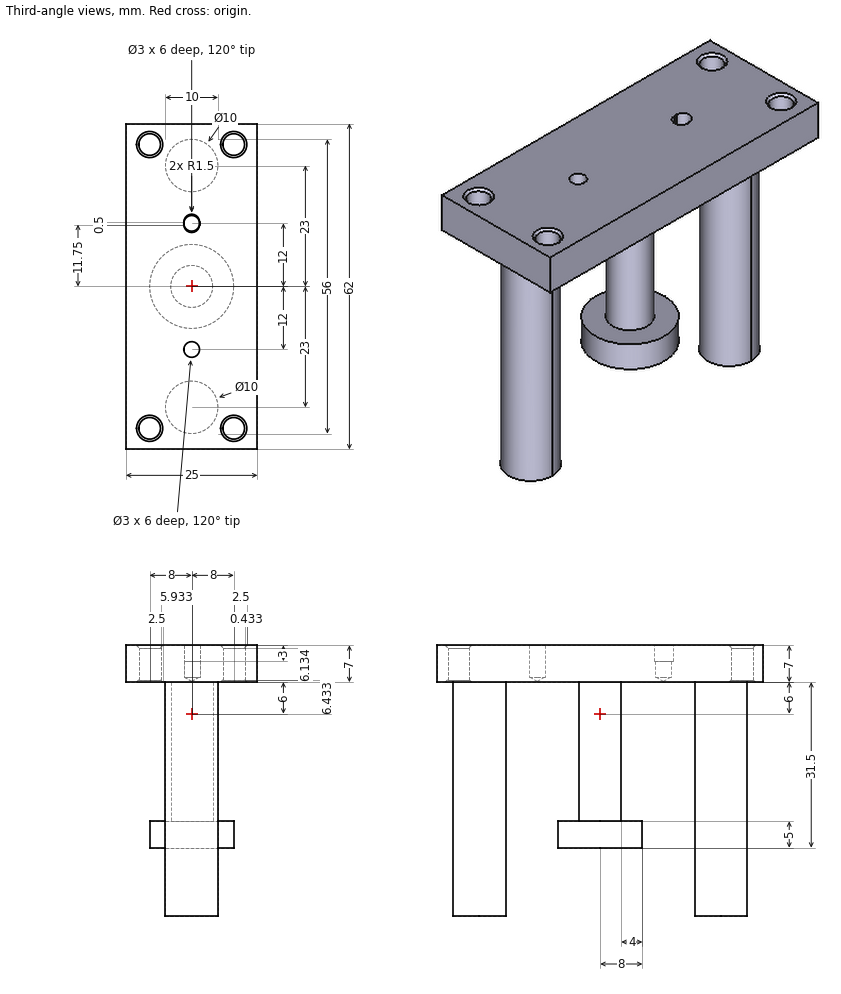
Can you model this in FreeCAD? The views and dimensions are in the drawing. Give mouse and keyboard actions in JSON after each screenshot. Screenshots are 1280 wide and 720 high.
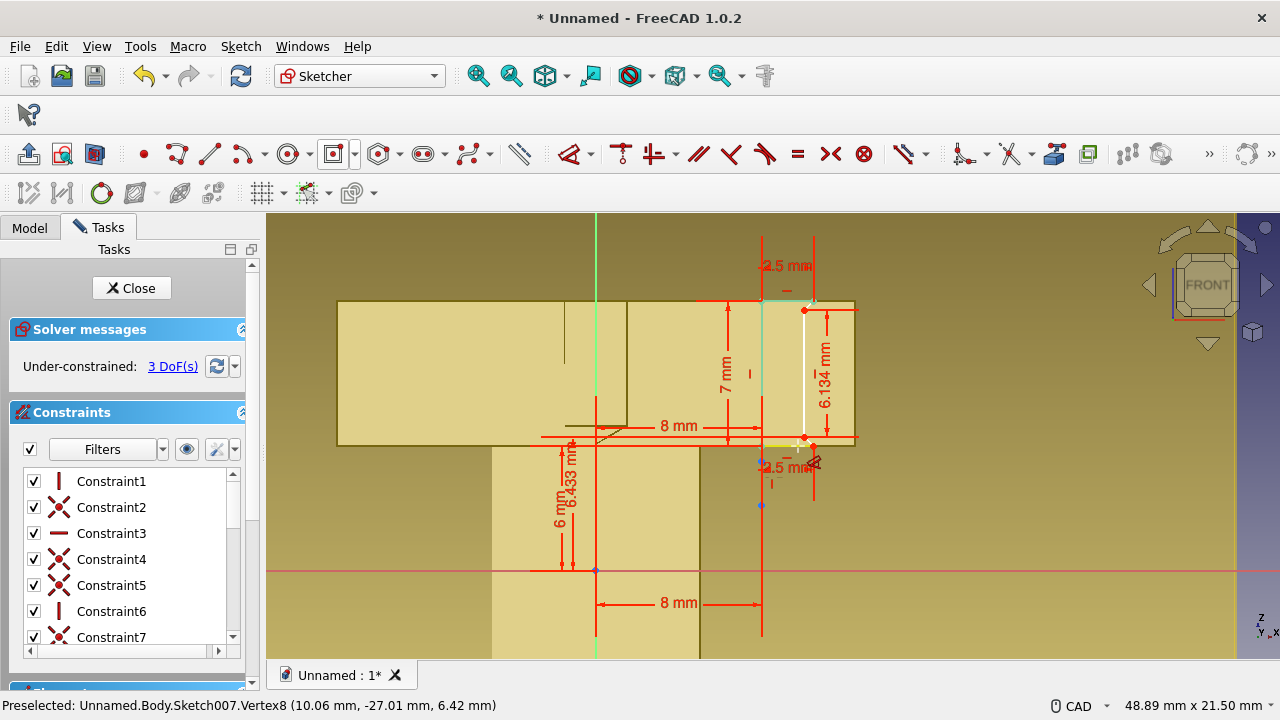
{"action": "scroll", "coordinate": [808, 307], "scroll_direction": "up", "scroll_amount": 8}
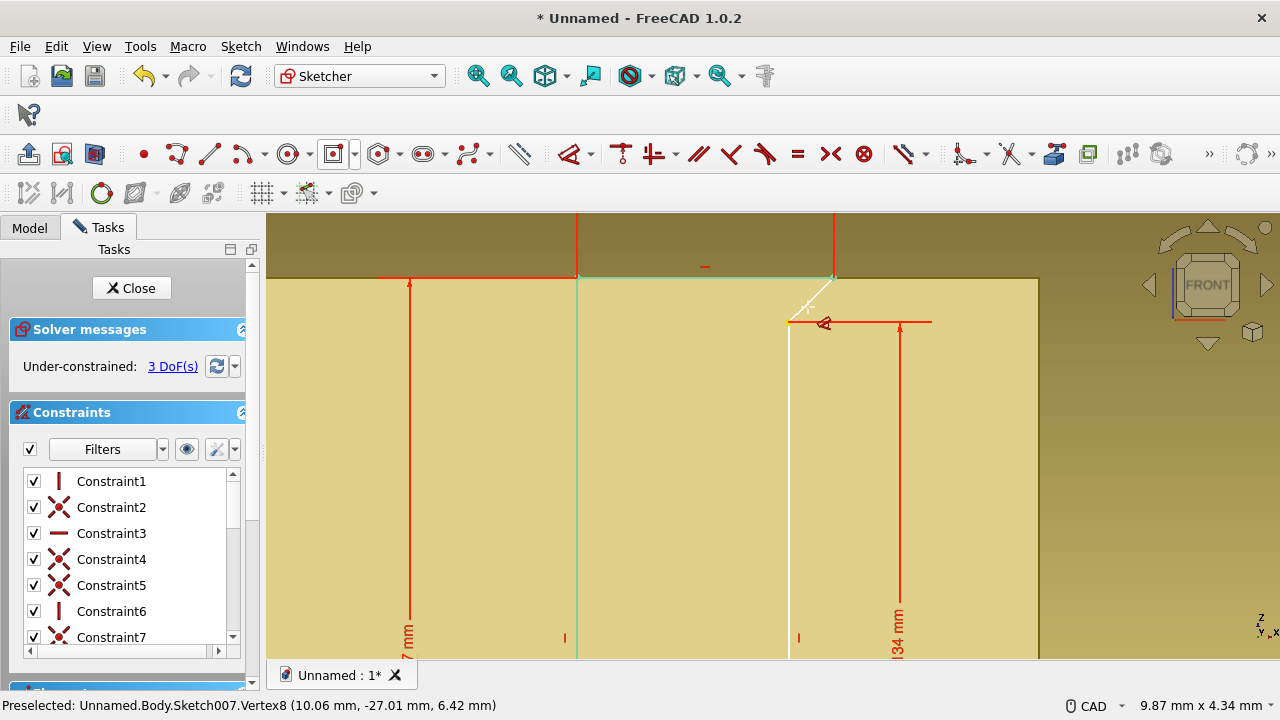
{"action": "left_click", "coordinate": [807, 305]}
{"action": "left_click", "coordinate": [811, 244]}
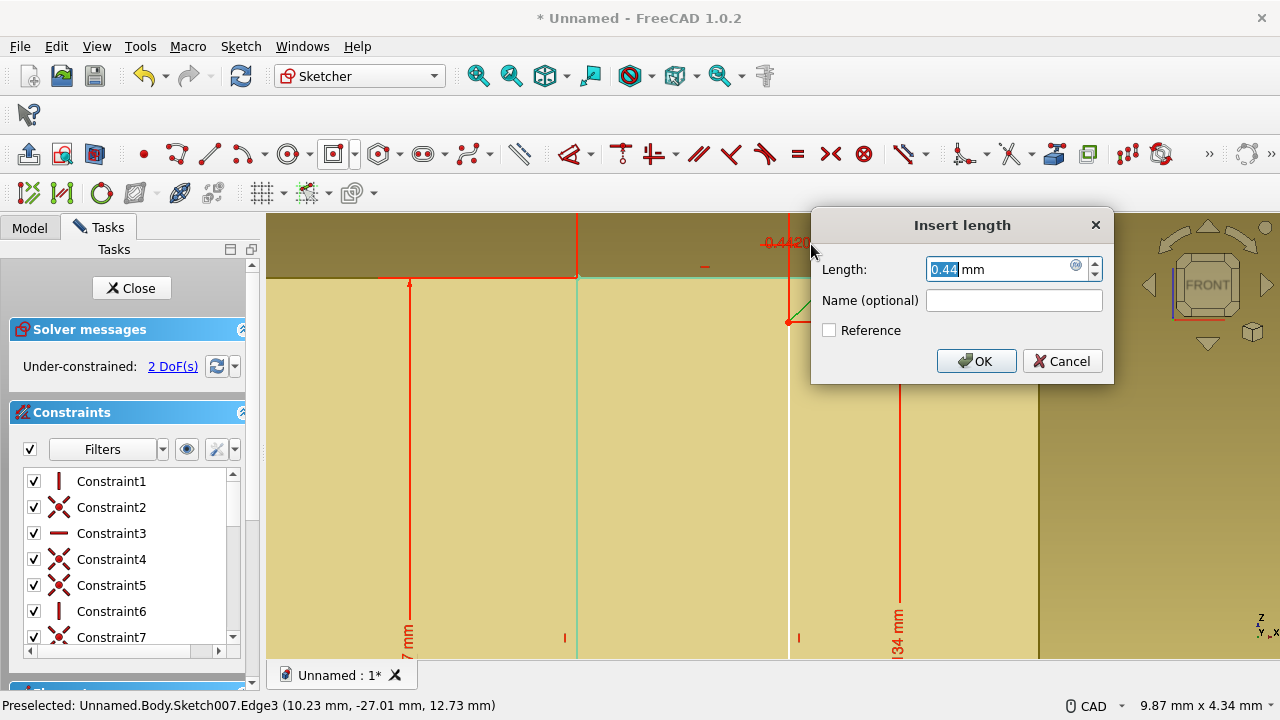
{"action": "type", "text": "0.433"}
{"action": "key", "text": "Return"}
{"action": "key", "text": "Escape"}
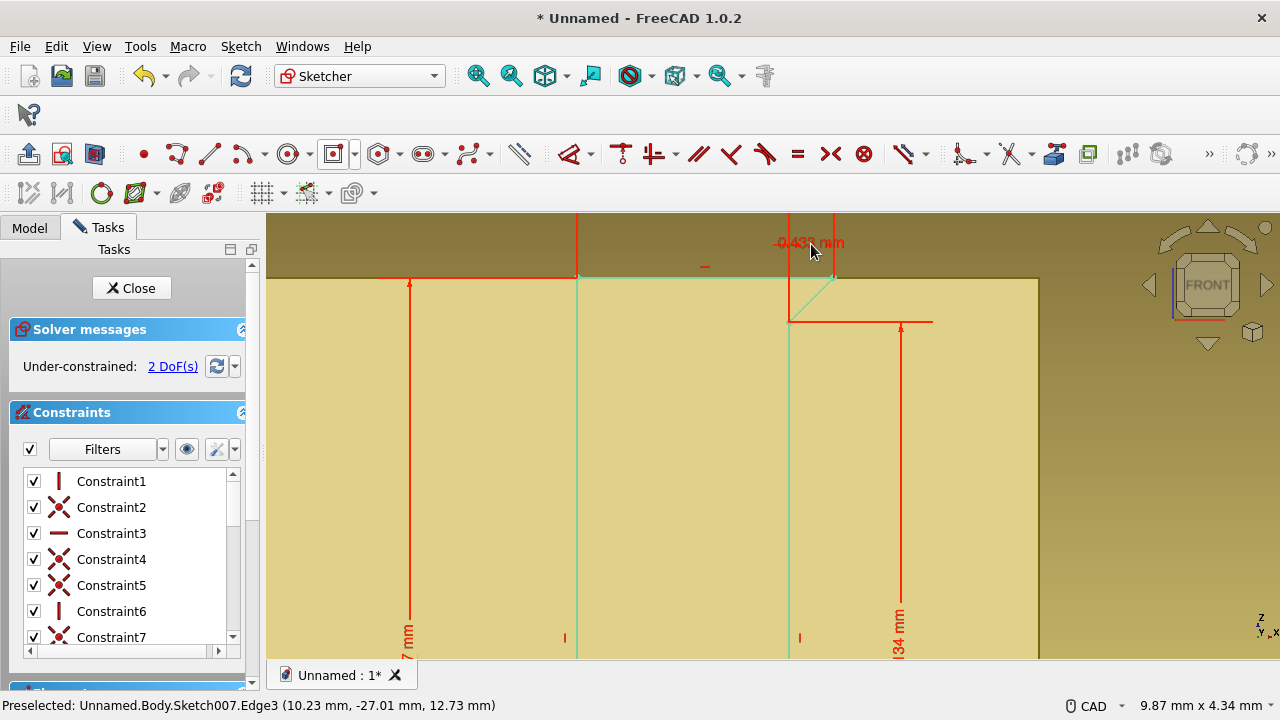
{"action": "left_click", "coordinate": [132, 288]}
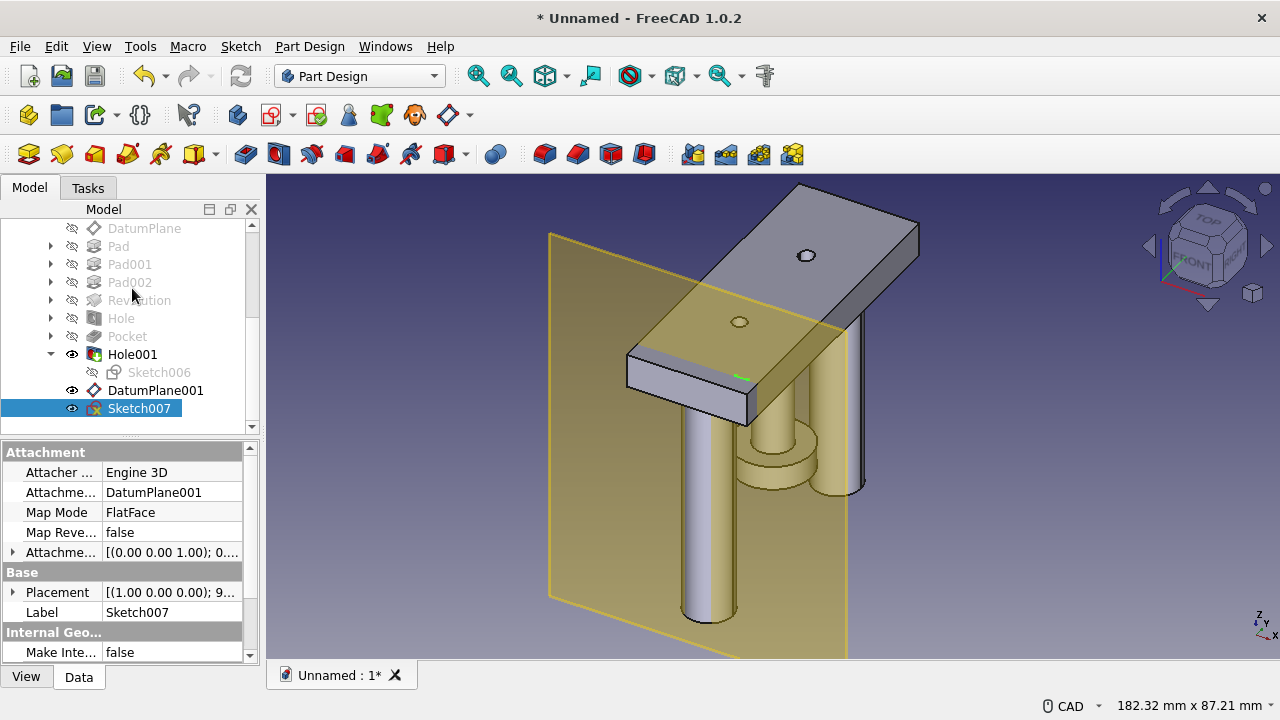
{"action": "left_click", "coordinate": [312, 154]}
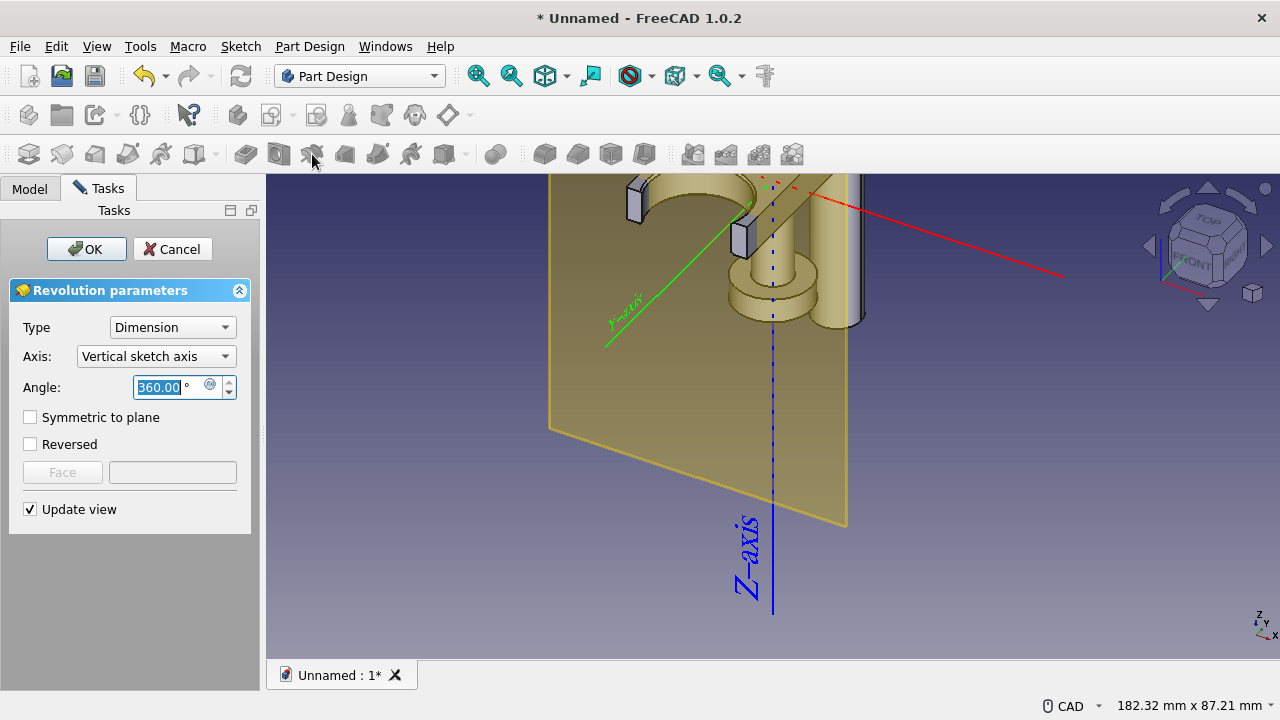
{"action": "left_click", "coordinate": [157, 356]}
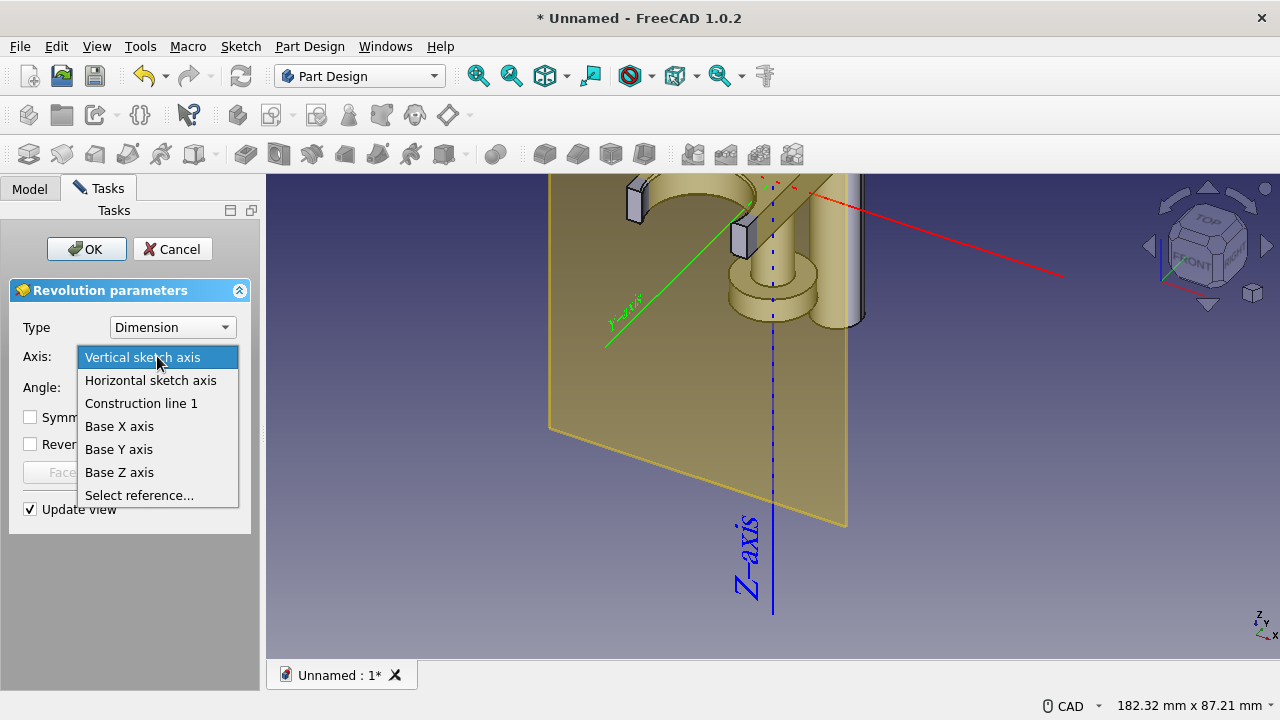
{"action": "left_click", "coordinate": [156, 404]}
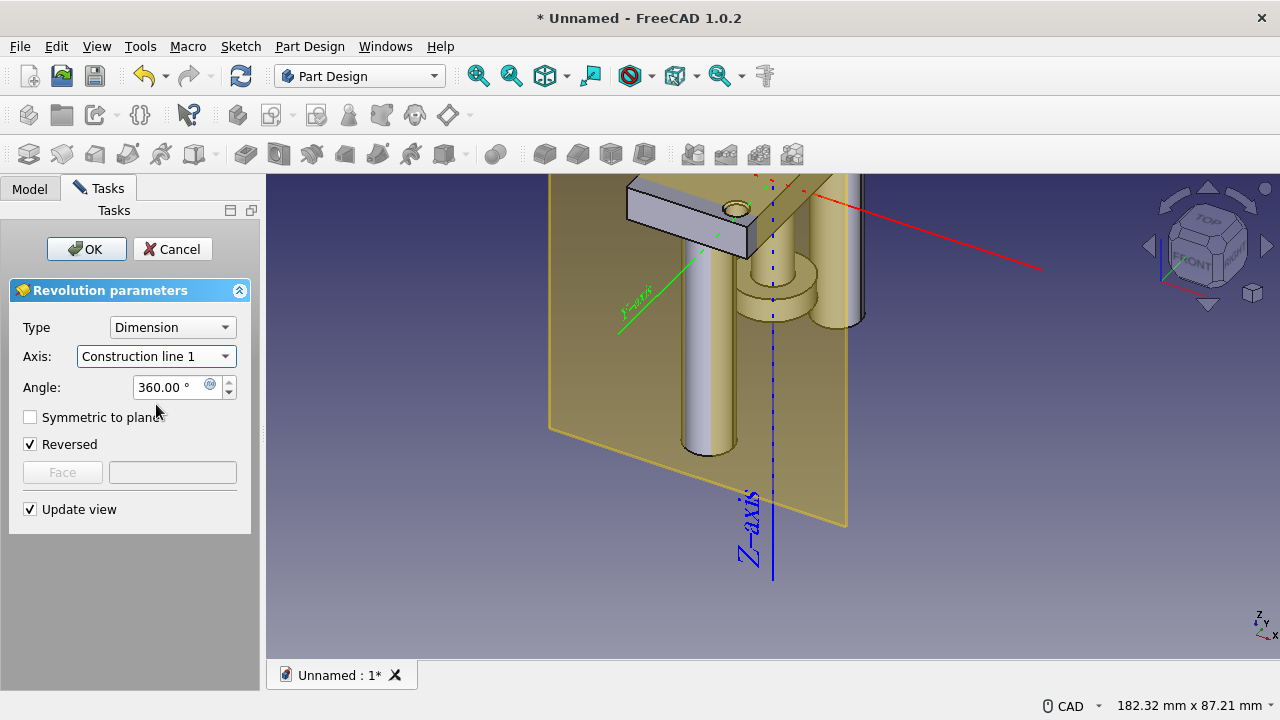
{"action": "left_click", "coordinate": [87, 249]}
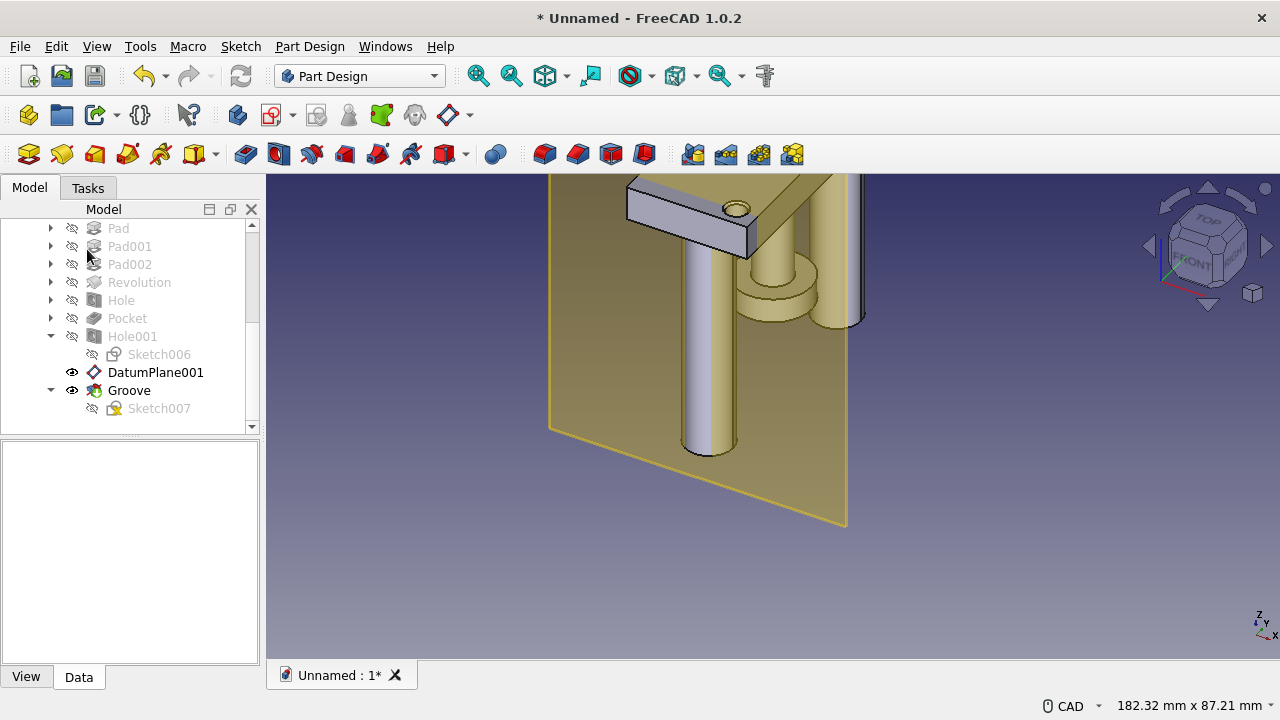
{"action": "left_click", "coordinate": [117, 372]}
{"action": "key", "text": "space"}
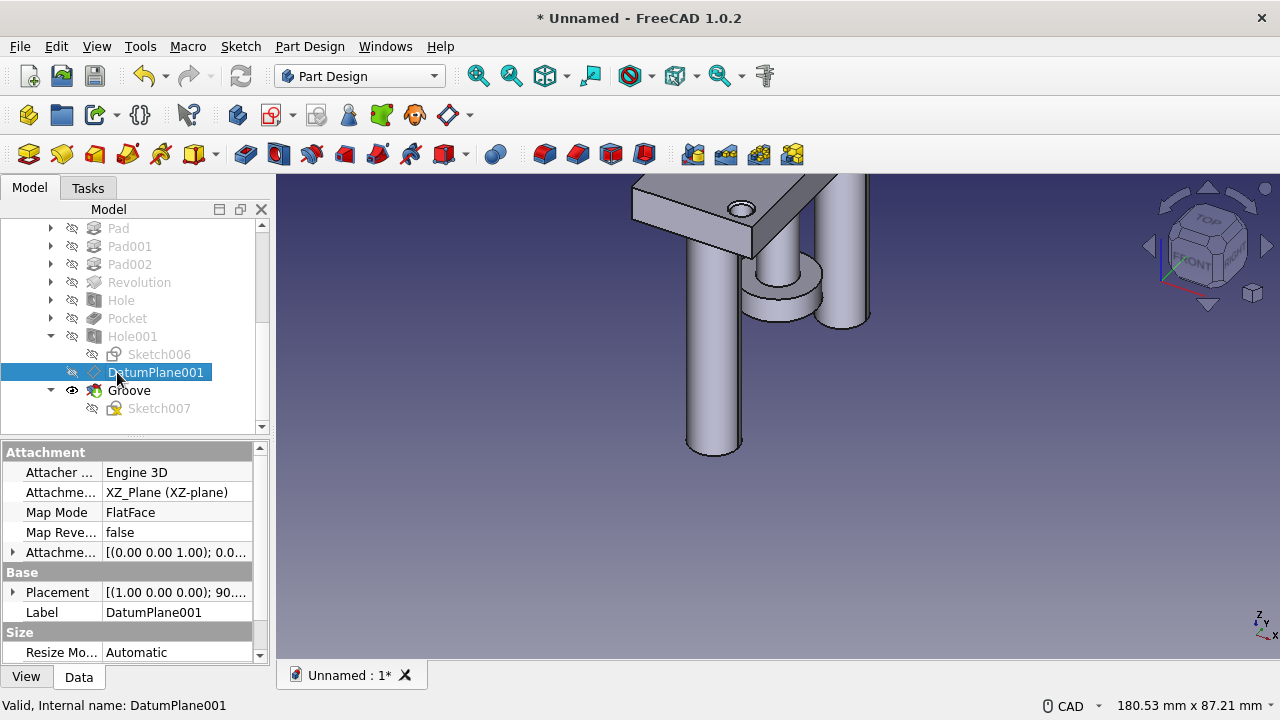
{"action": "left_click", "coordinate": [479, 76]}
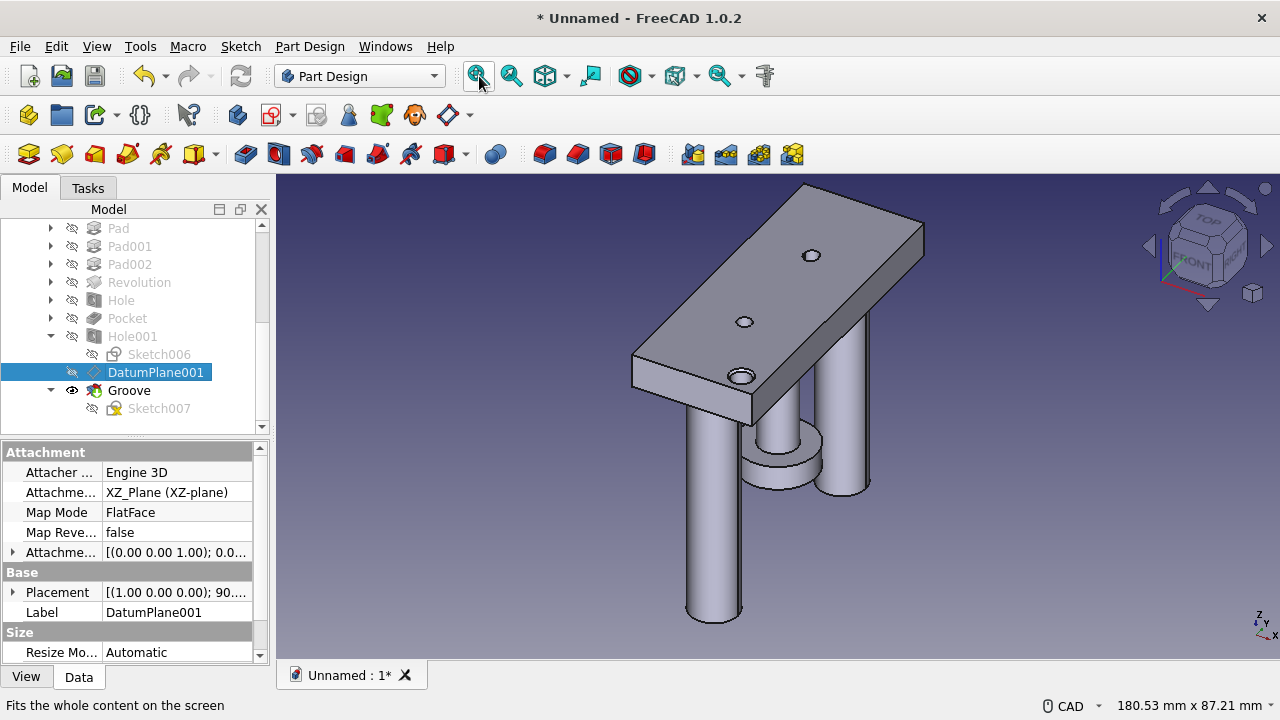
{"action": "scroll", "coordinate": [141, 314], "scroll_direction": "down", "scroll_amount": 3}